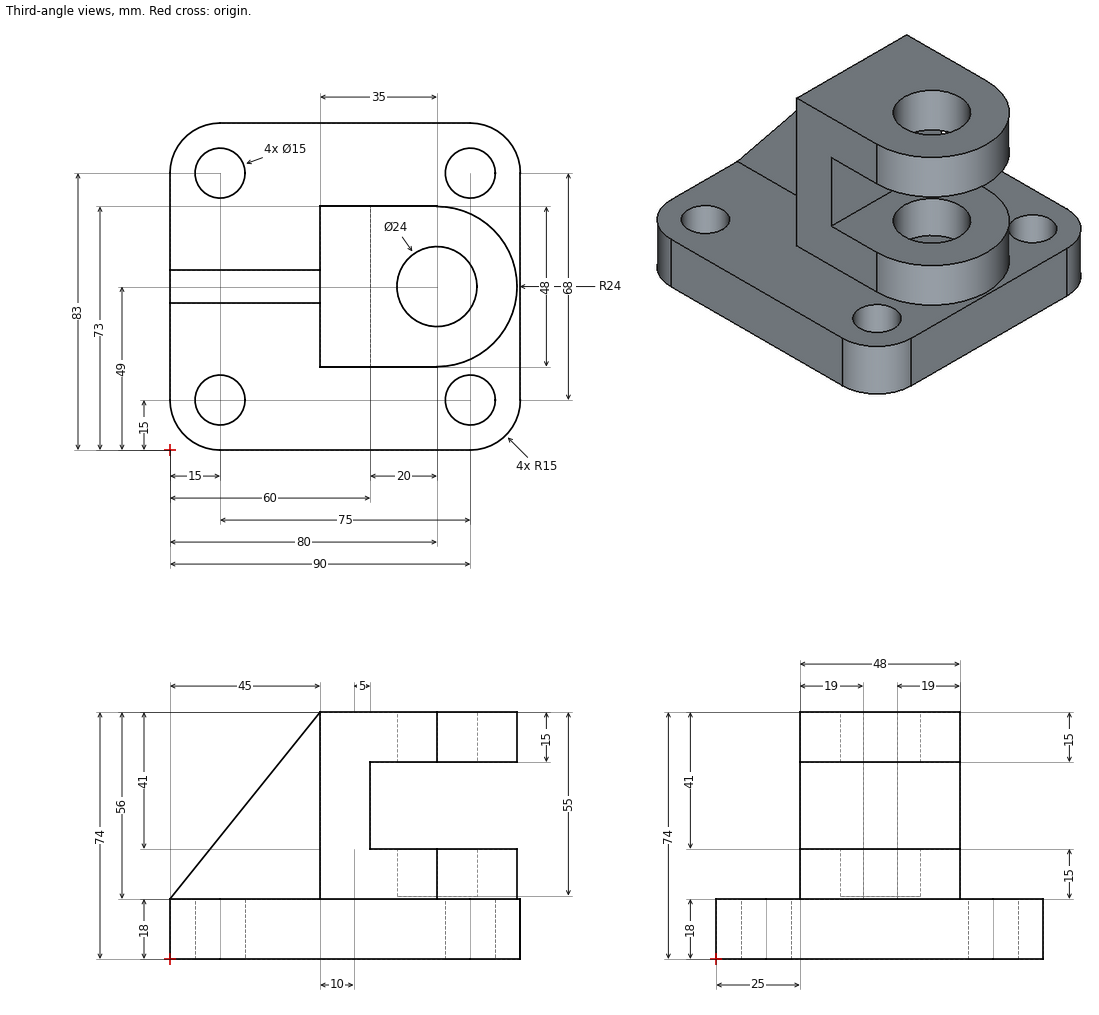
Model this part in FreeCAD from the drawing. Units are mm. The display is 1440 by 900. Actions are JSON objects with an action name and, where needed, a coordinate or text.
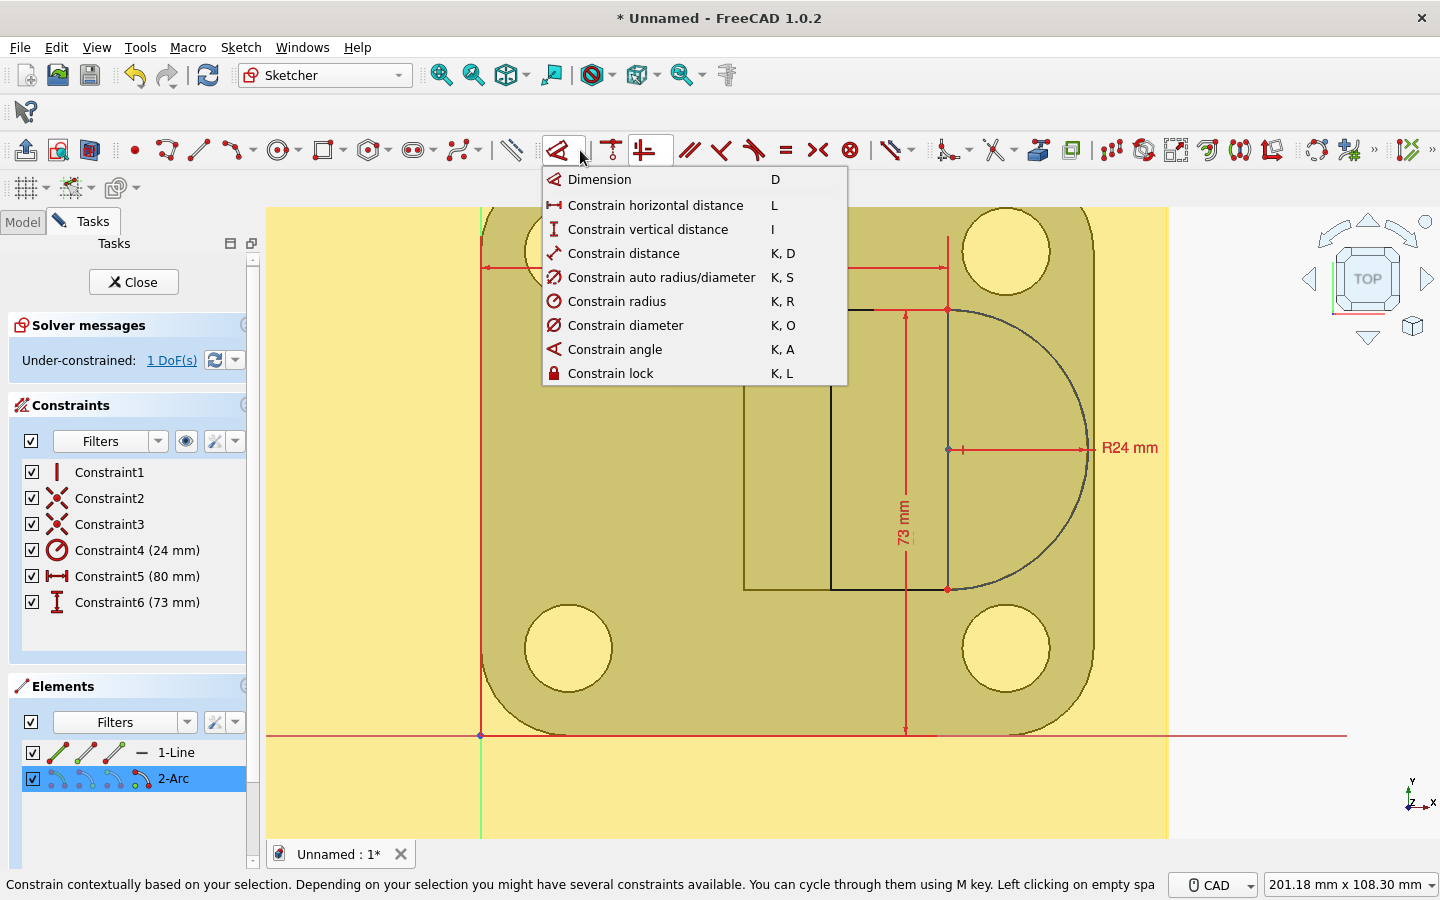
{"action": "left_click", "coordinate": [695, 205]}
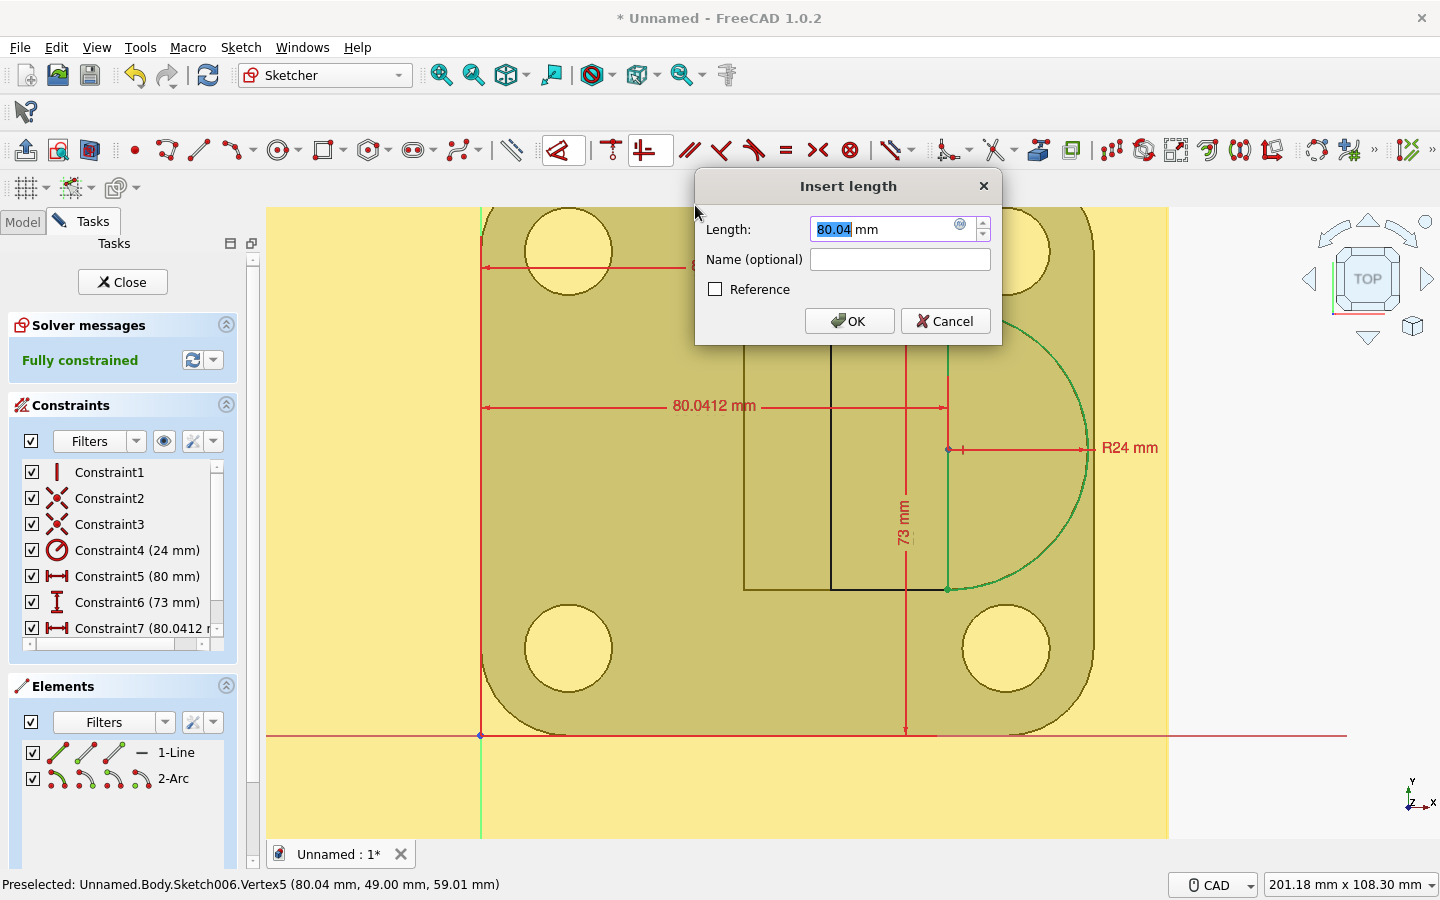
{"action": "type", "text": "80"}
{"action": "key", "text": "Return"}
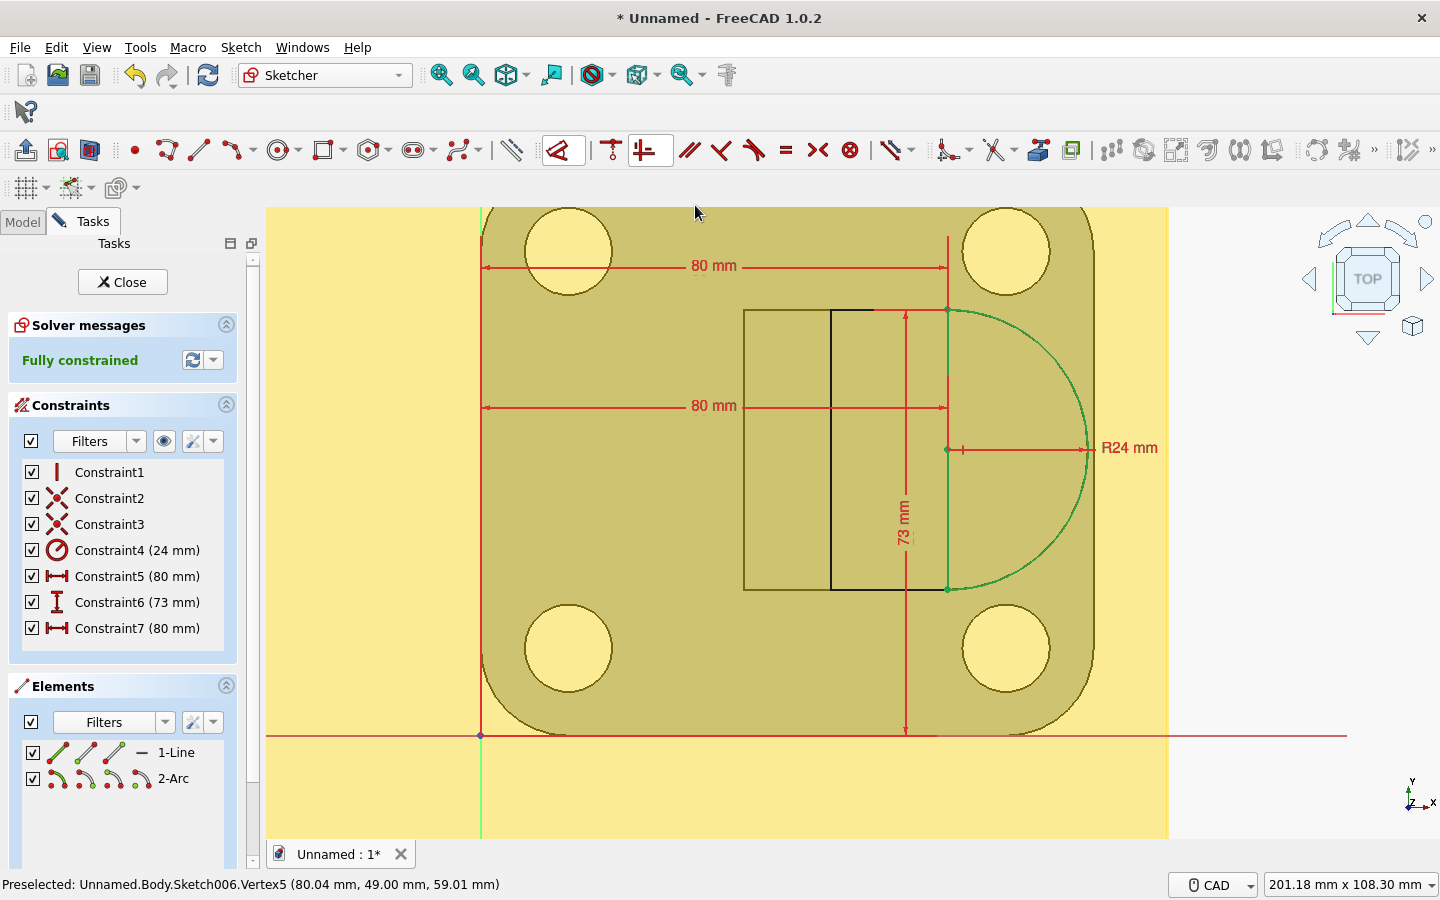
{"action": "left_click", "coordinate": [123, 282]}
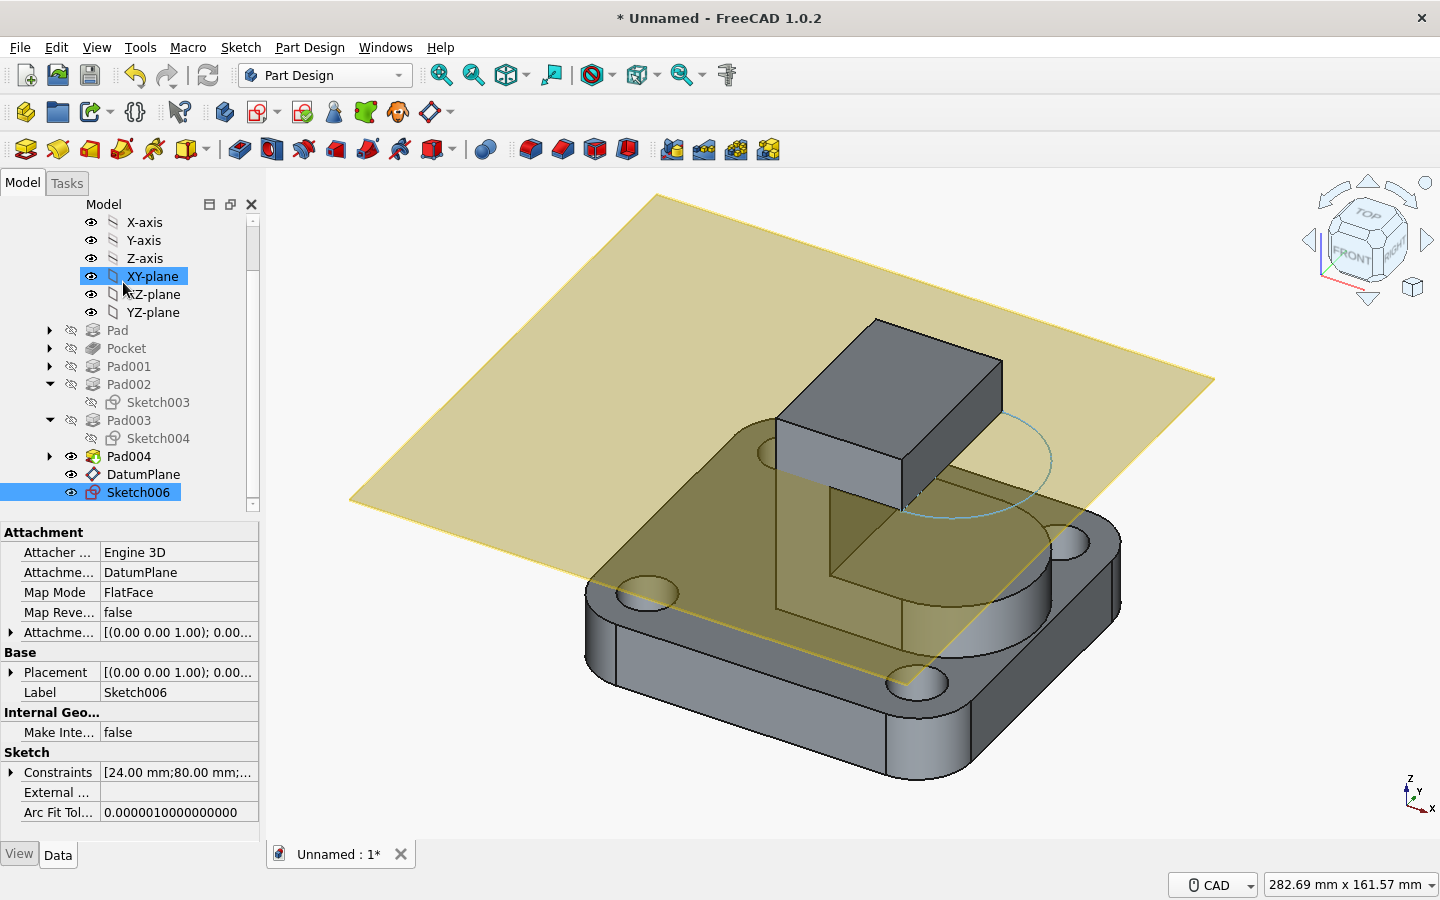
{"action": "left_click", "coordinate": [26, 150]}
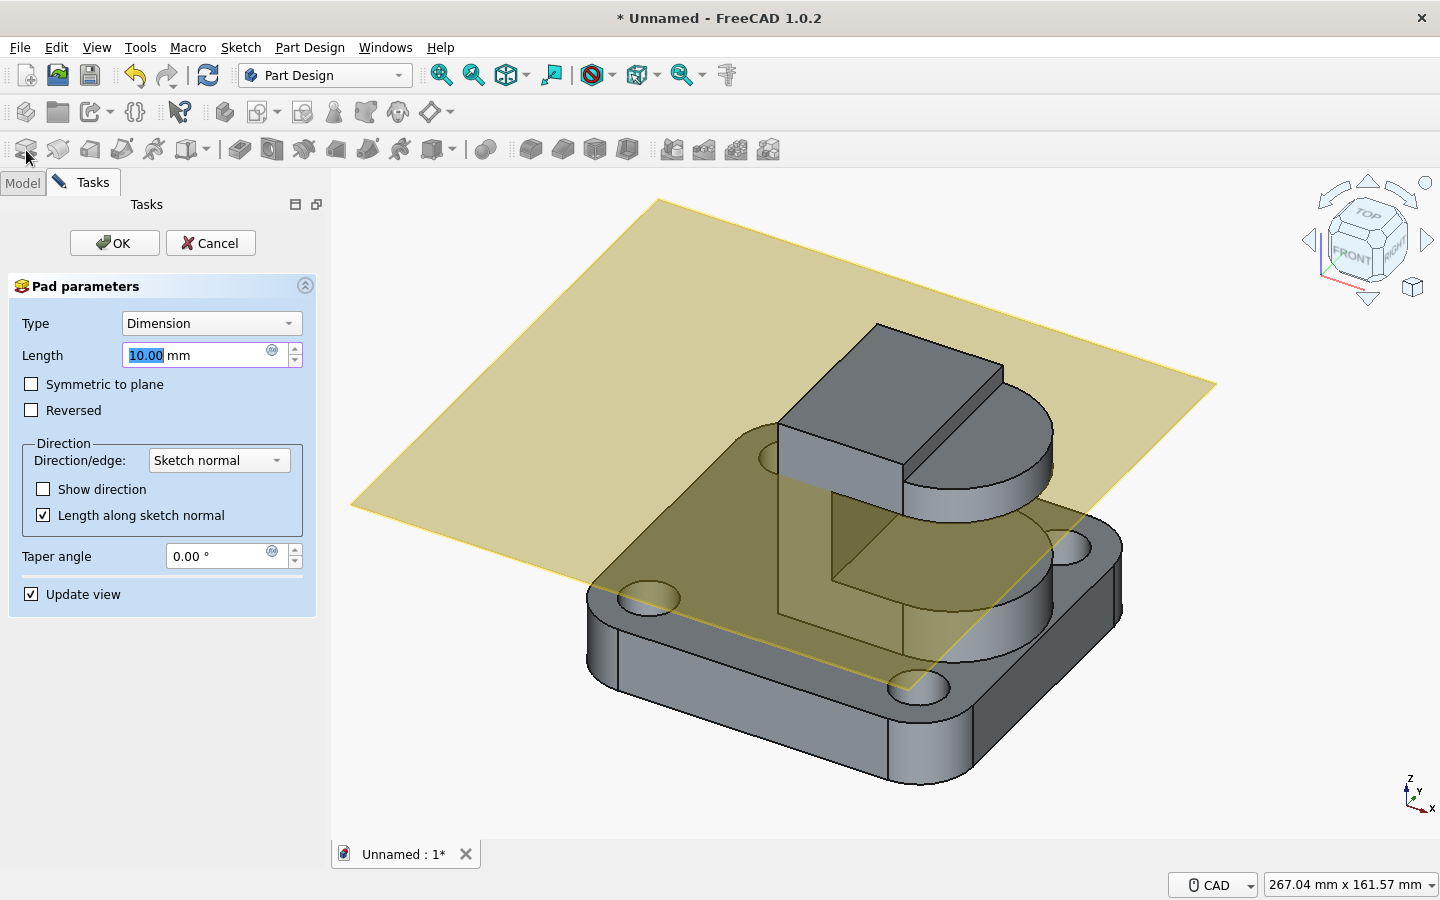
{"action": "type", "text": "15"}
{"action": "key", "text": "Tab"}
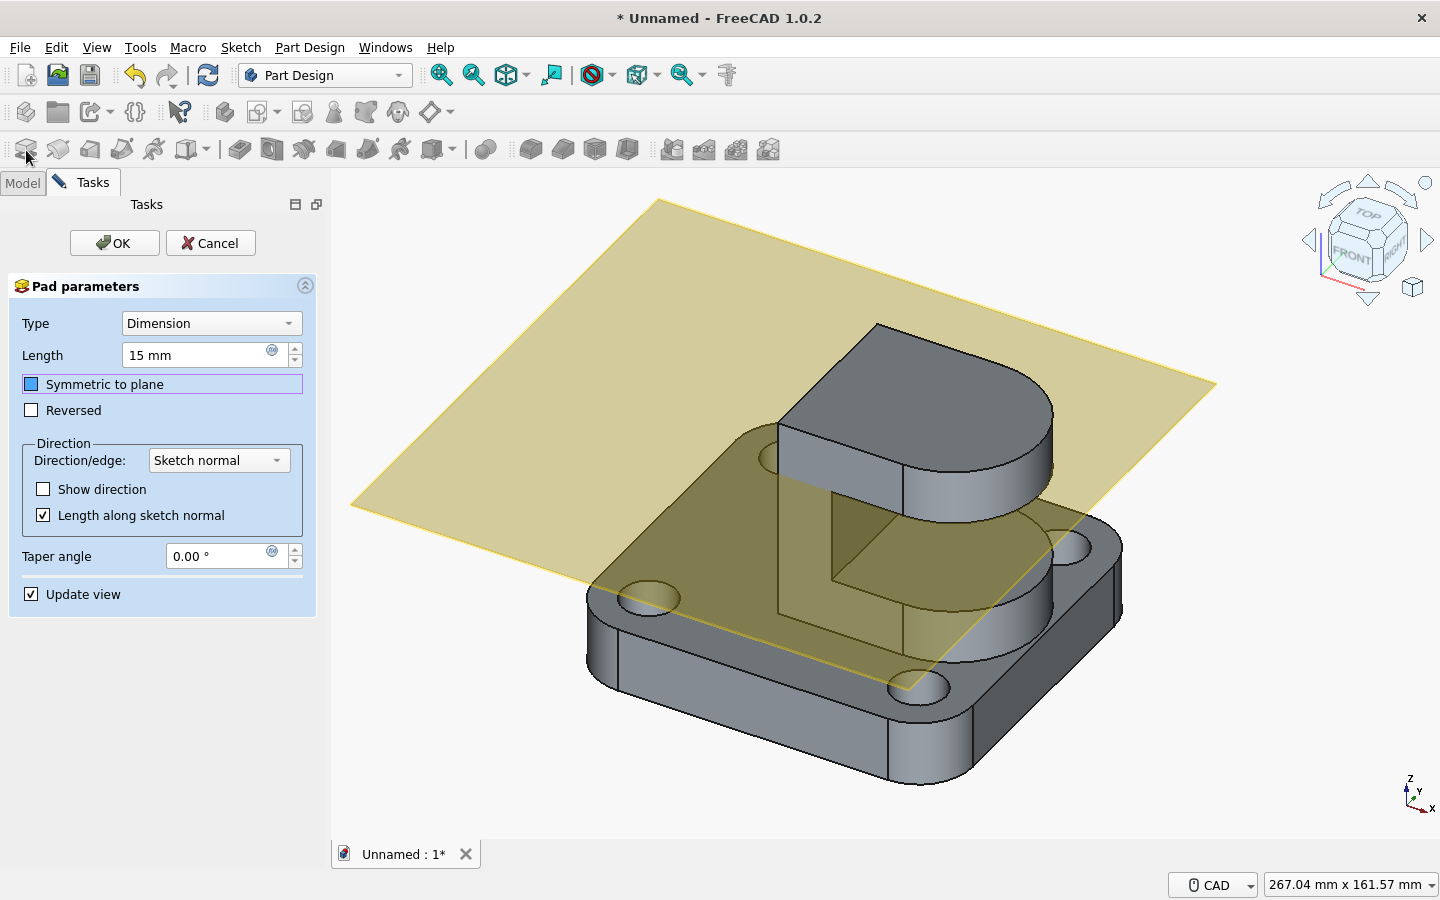
{"action": "left_click", "coordinate": [115, 243]}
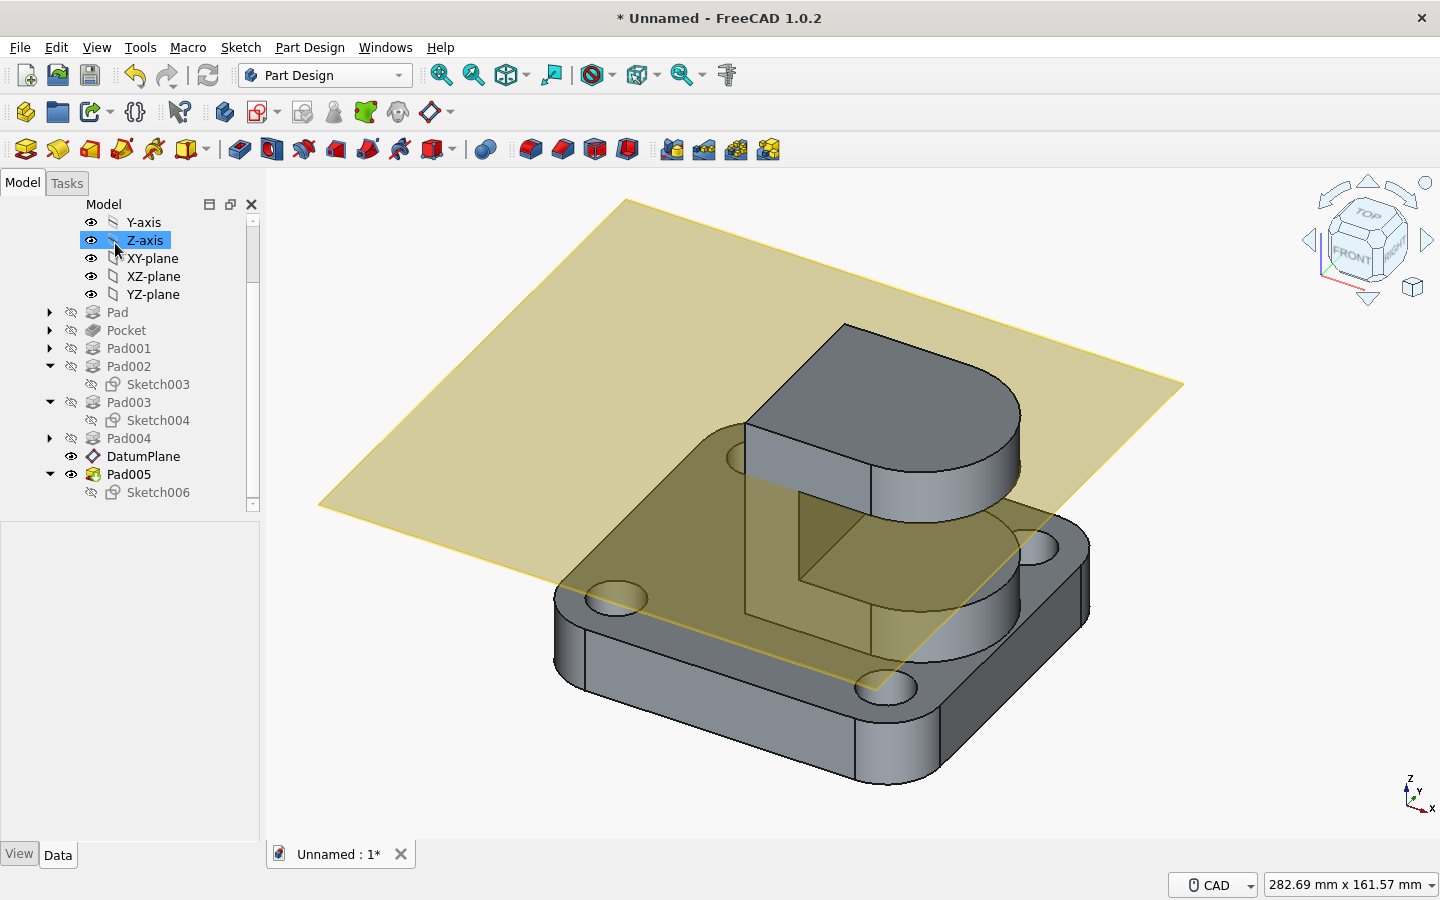
{"action": "left_click", "coordinate": [116, 456]}
{"action": "key", "text": "space"}